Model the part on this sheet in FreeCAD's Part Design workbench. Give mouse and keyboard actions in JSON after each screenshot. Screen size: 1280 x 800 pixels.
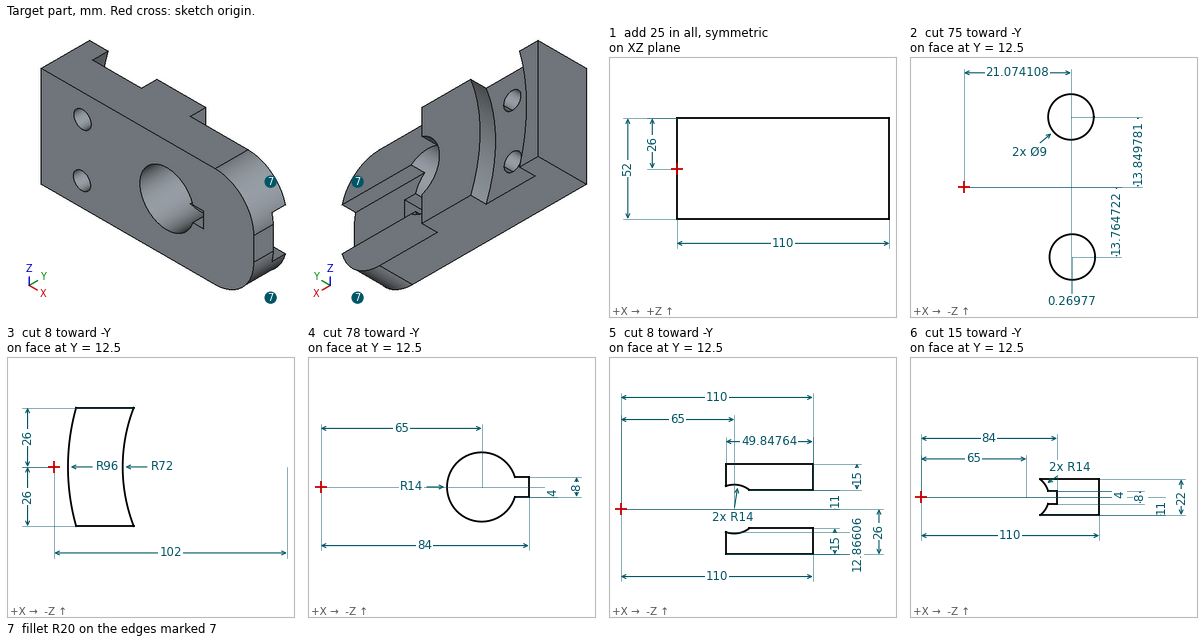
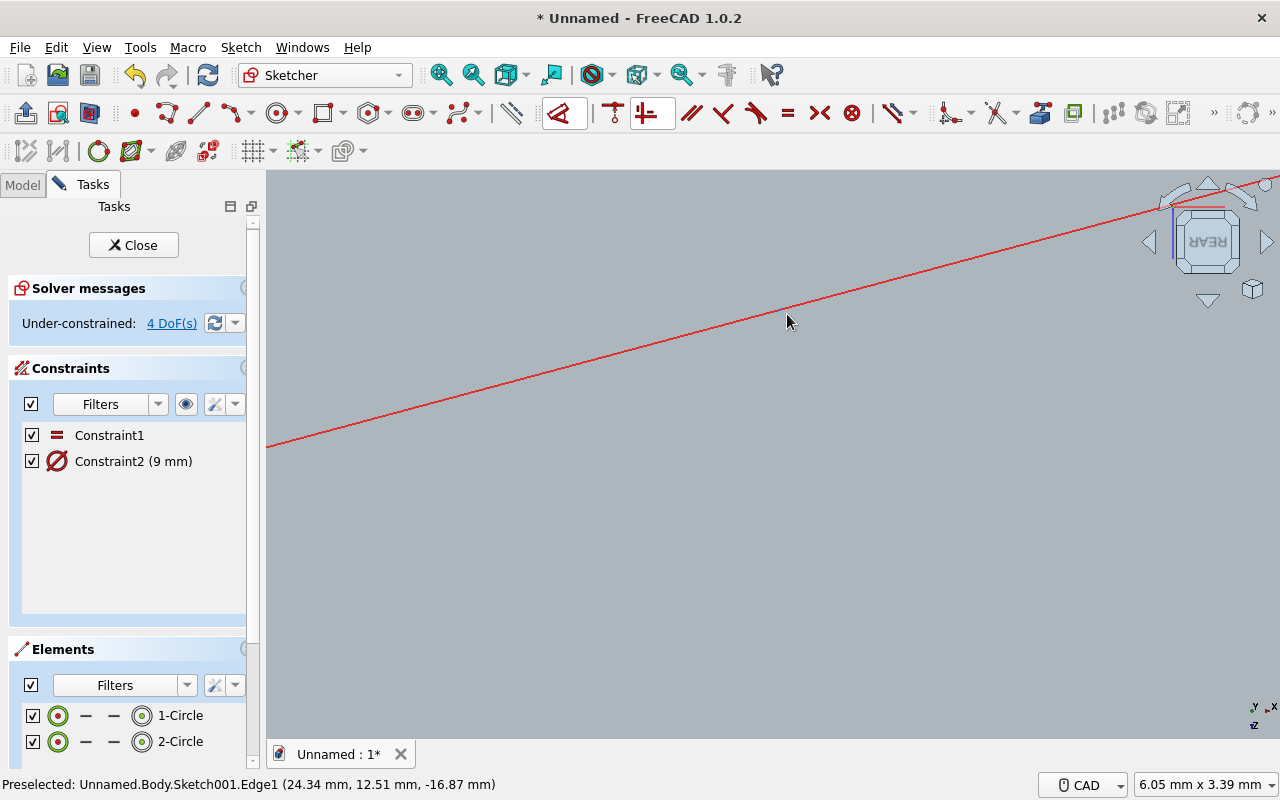
{"action": "left_click", "coordinate": [779, 310]}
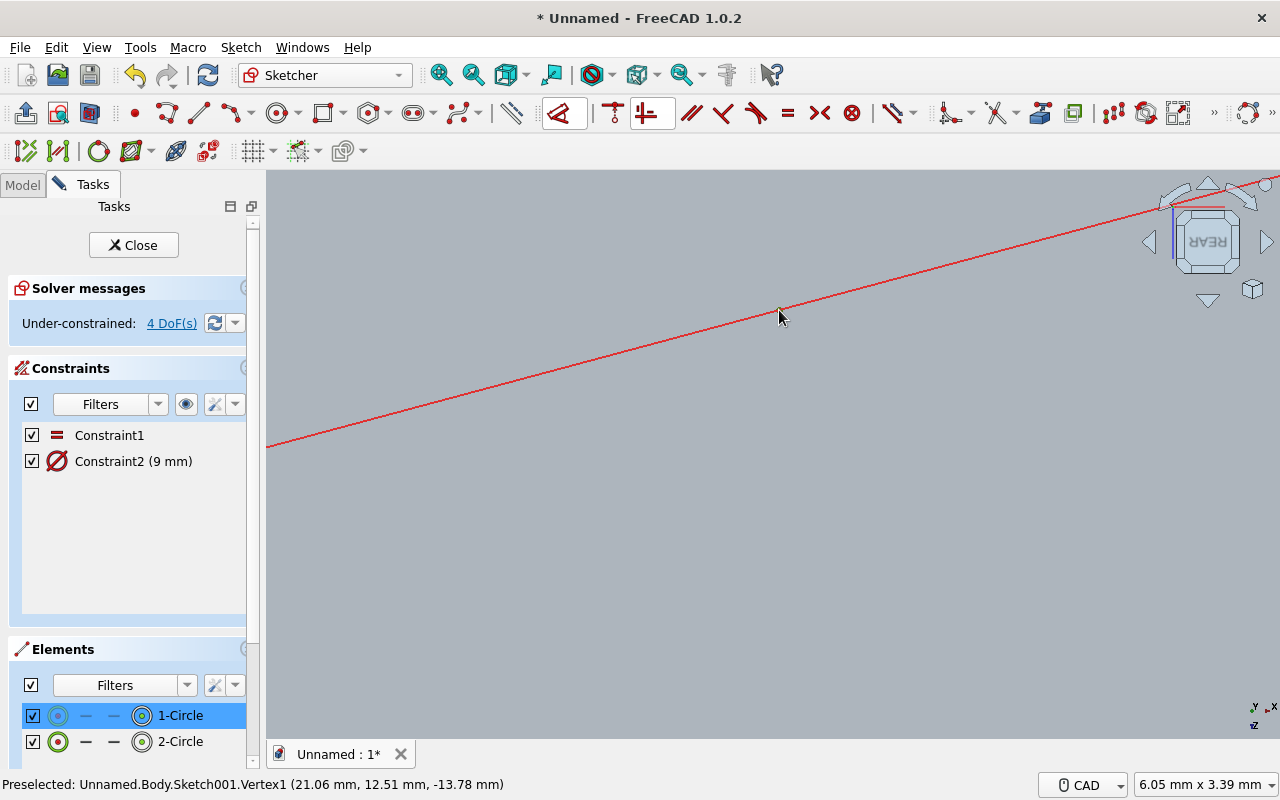
{"action": "scroll", "coordinate": [788, 315], "scroll_direction": "down", "scroll_amount": 14}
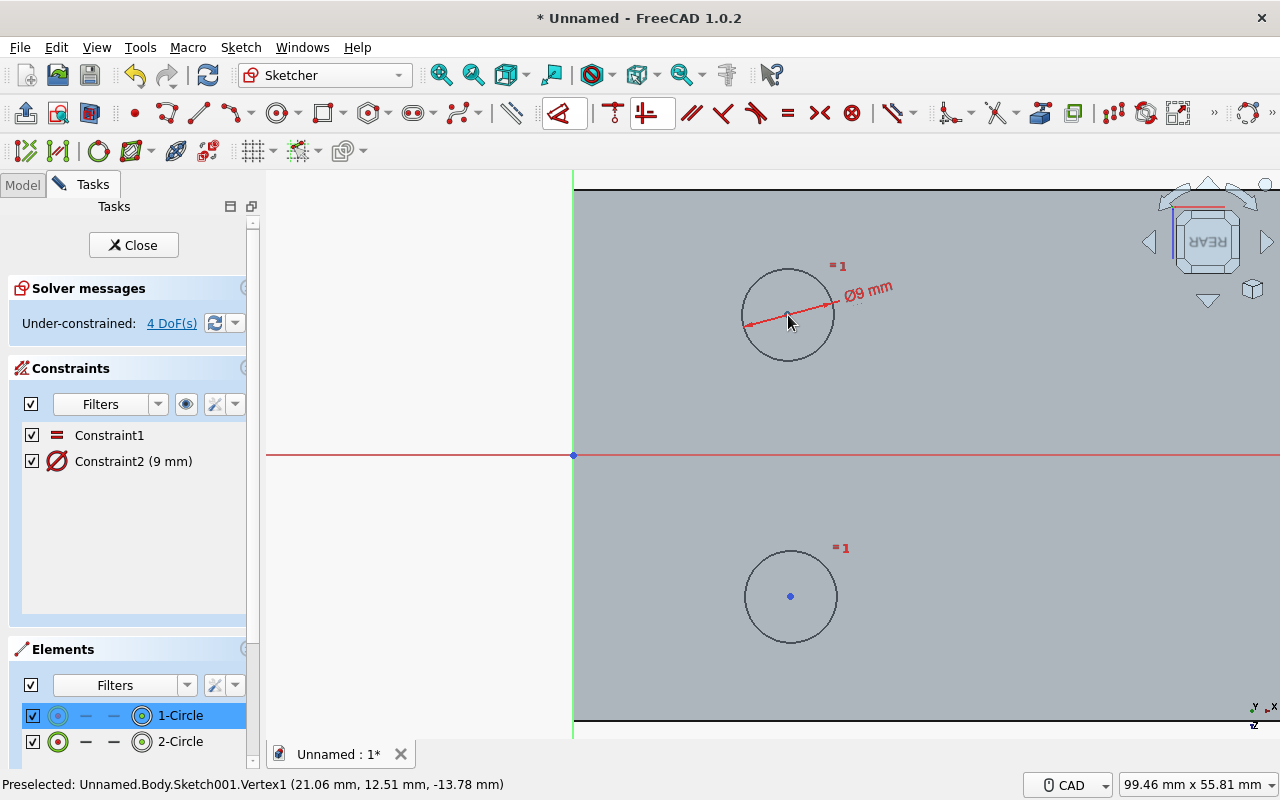
{"action": "scroll", "coordinate": [791, 597], "scroll_direction": "up", "scroll_amount": 14}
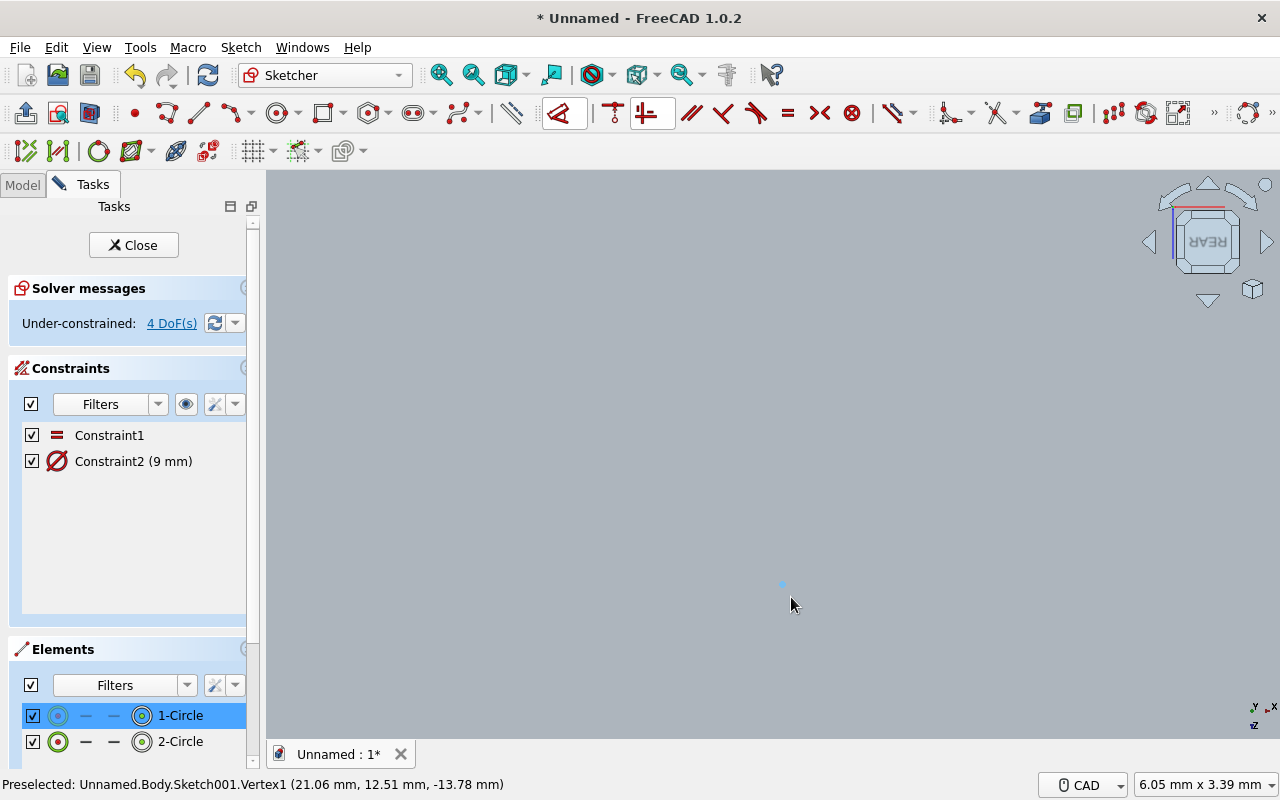
{"action": "left_click", "coordinate": [782, 584]}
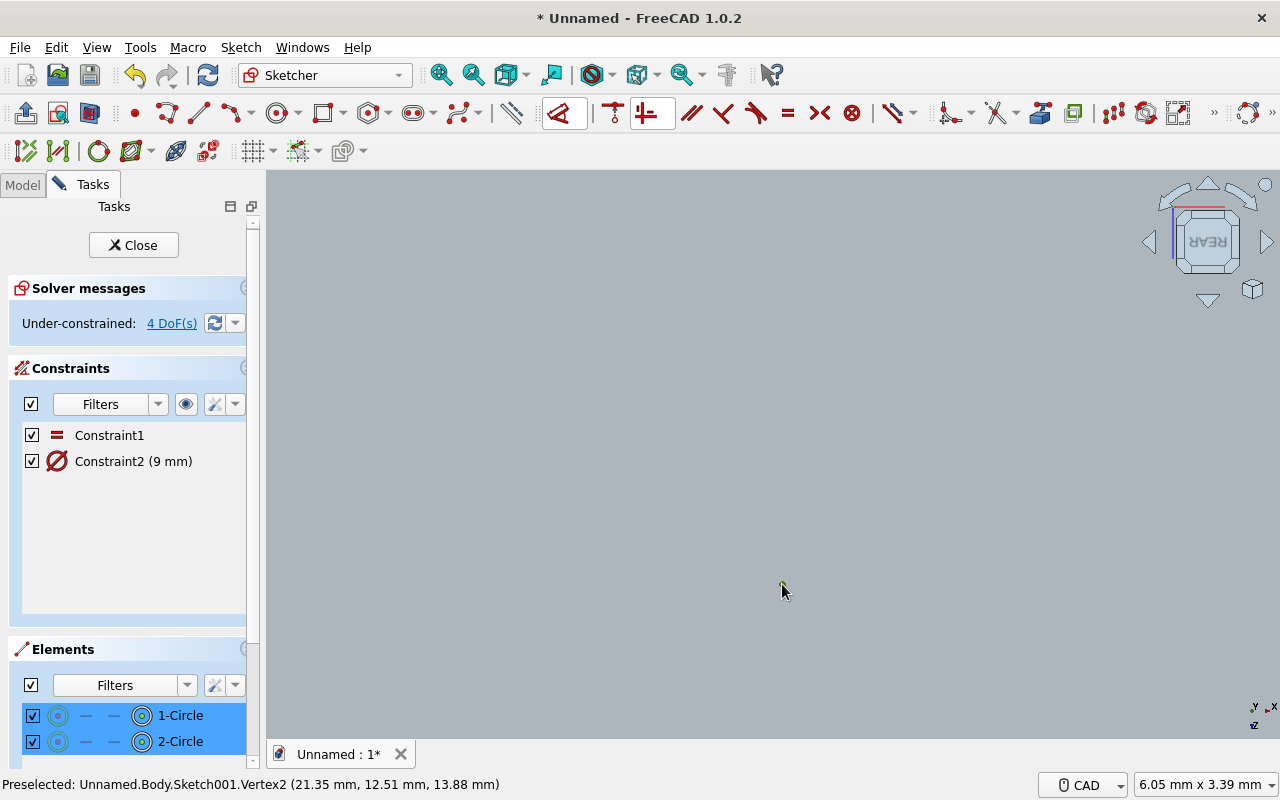
{"action": "left_click", "coordinate": [582, 114]}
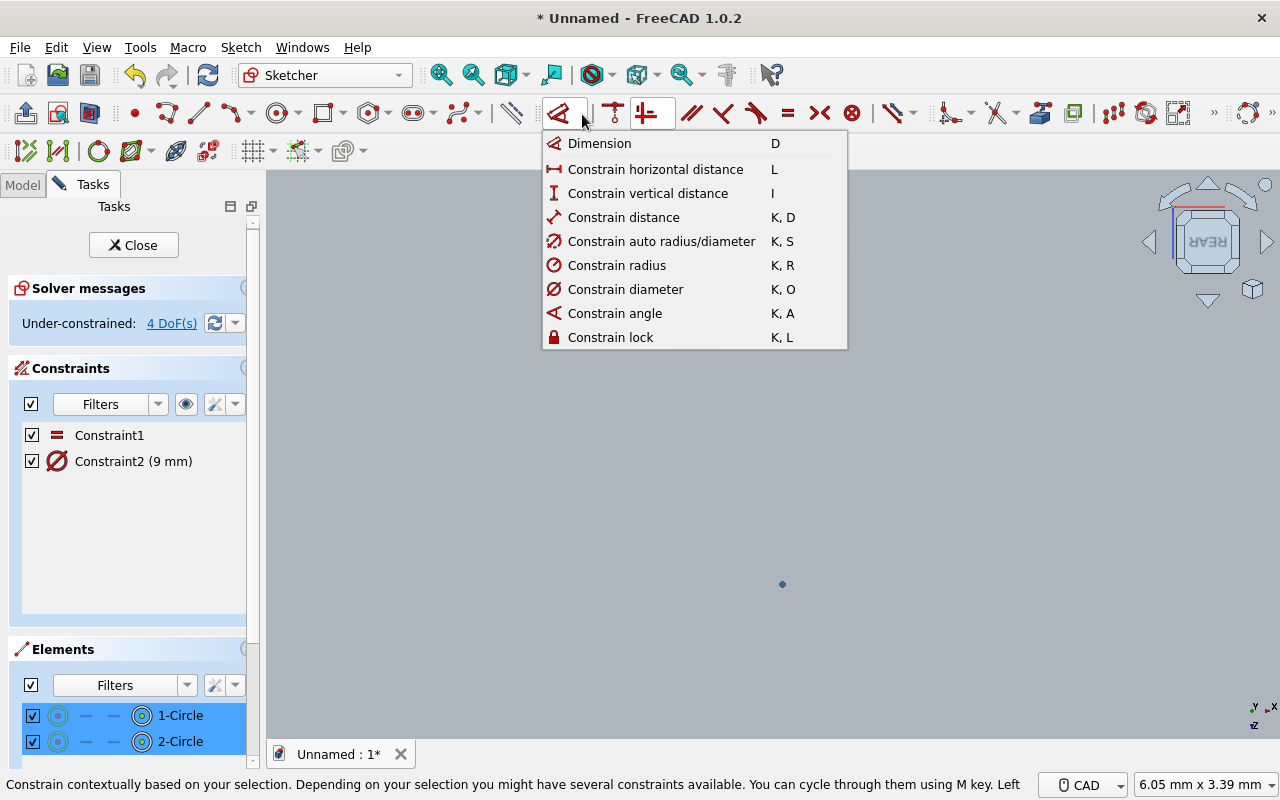
{"action": "left_click", "coordinate": [695, 169]}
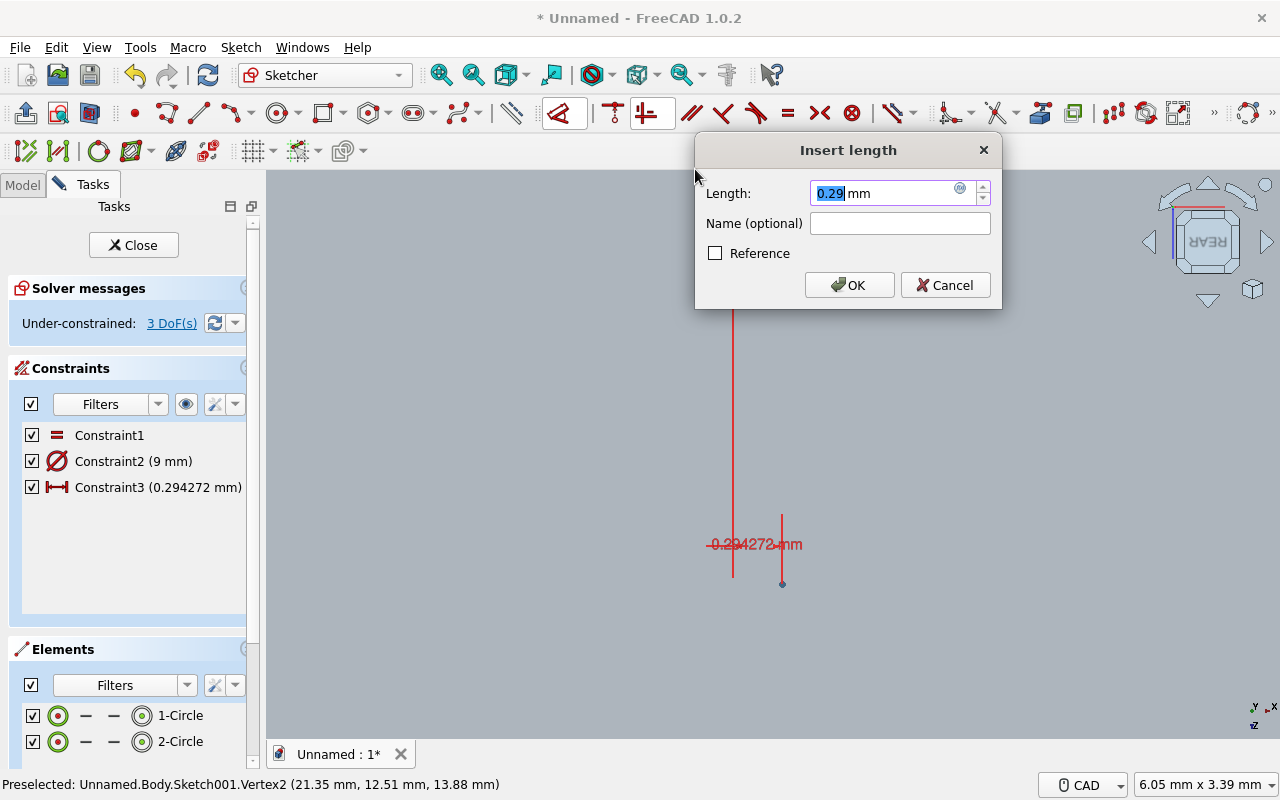
{"action": "type", "text": "0.26977"}
{"action": "key", "text": "Return"}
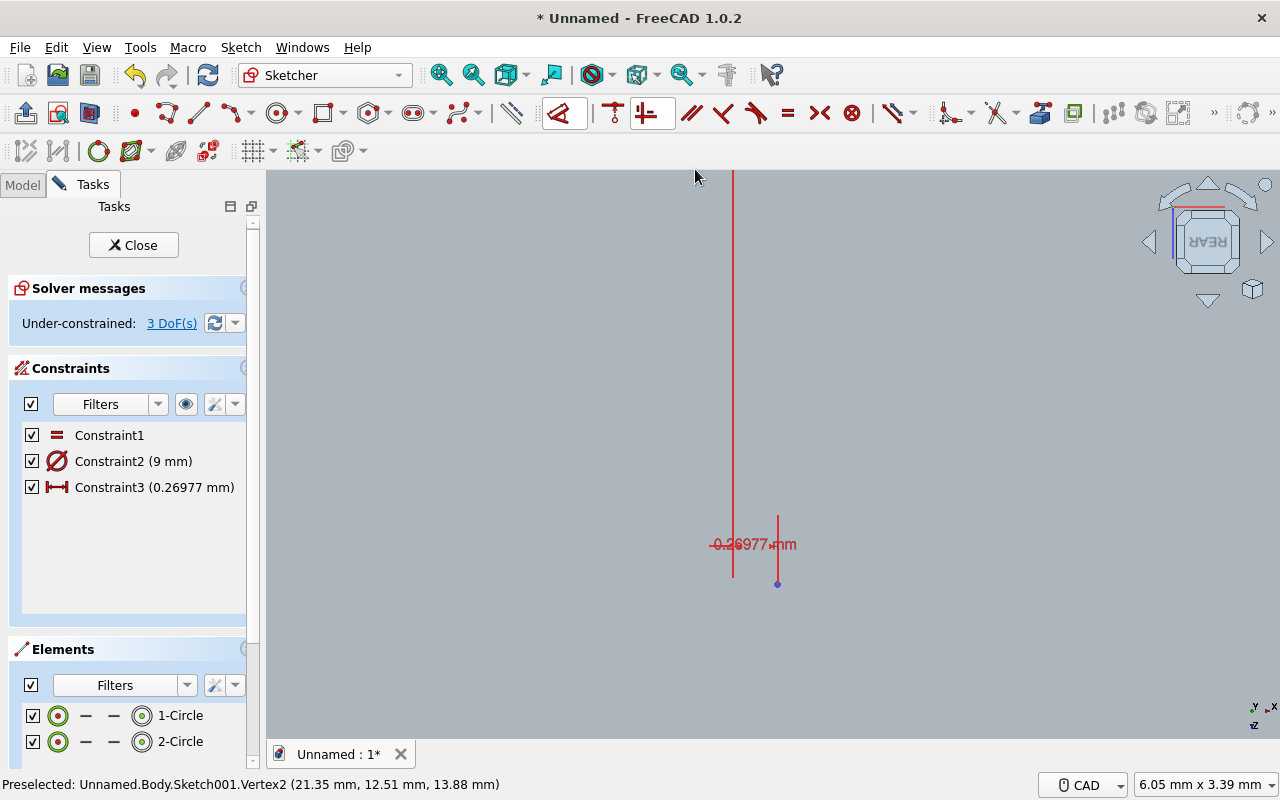
{"action": "scroll", "coordinate": [791, 597], "scroll_direction": "down", "scroll_amount": 14}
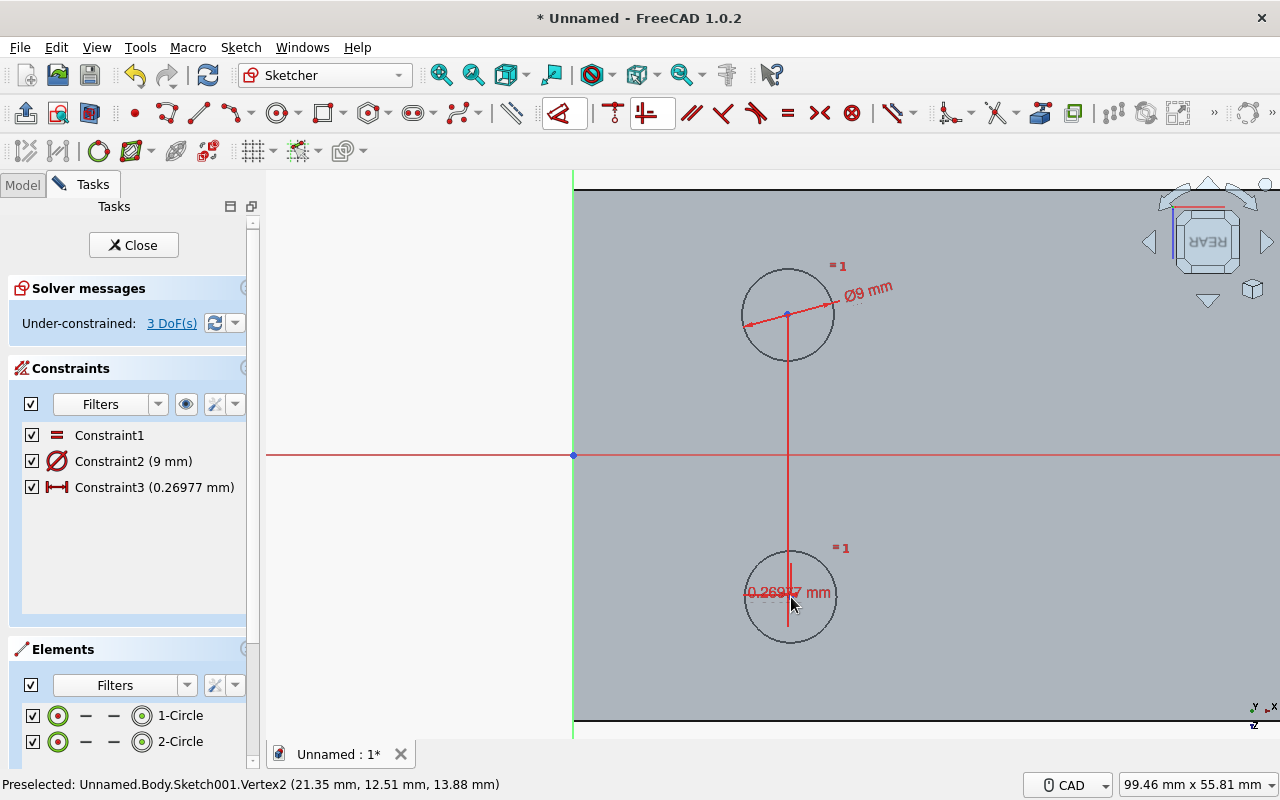
{"action": "left_click", "coordinate": [788, 315]}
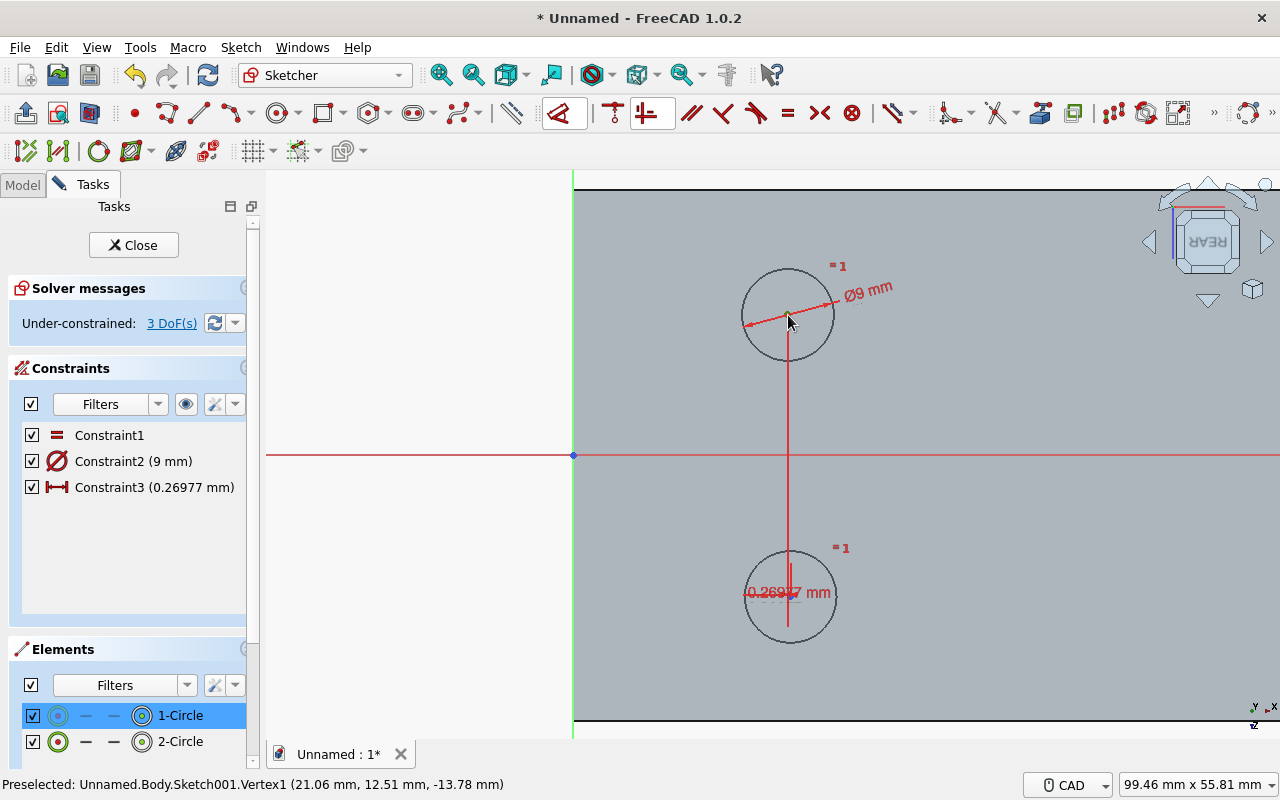
{"action": "key", "text": "l"}